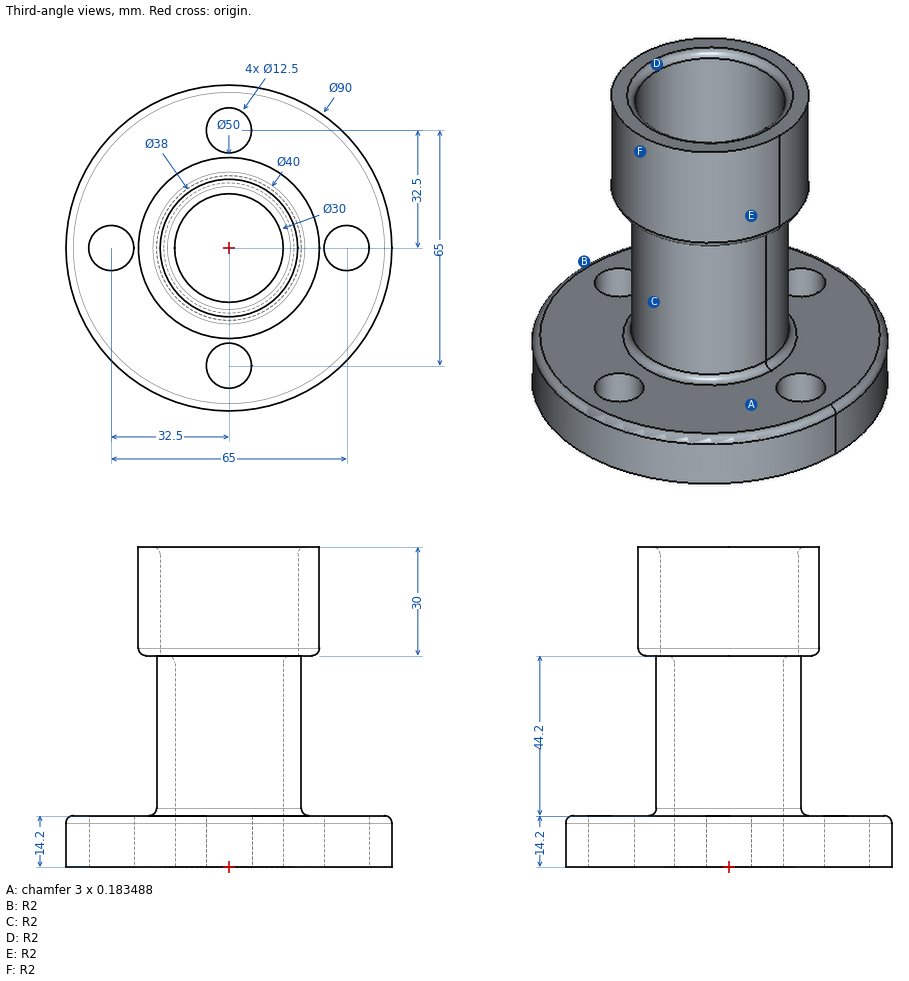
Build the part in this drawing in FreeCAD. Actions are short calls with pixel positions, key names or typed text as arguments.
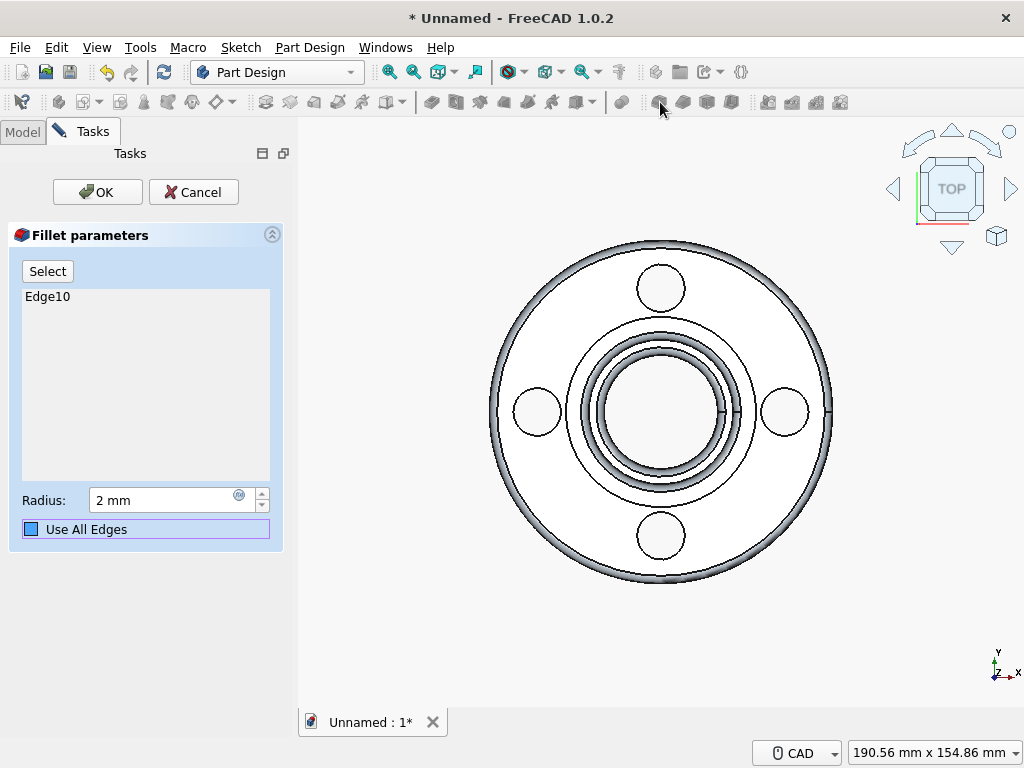
click(98, 192)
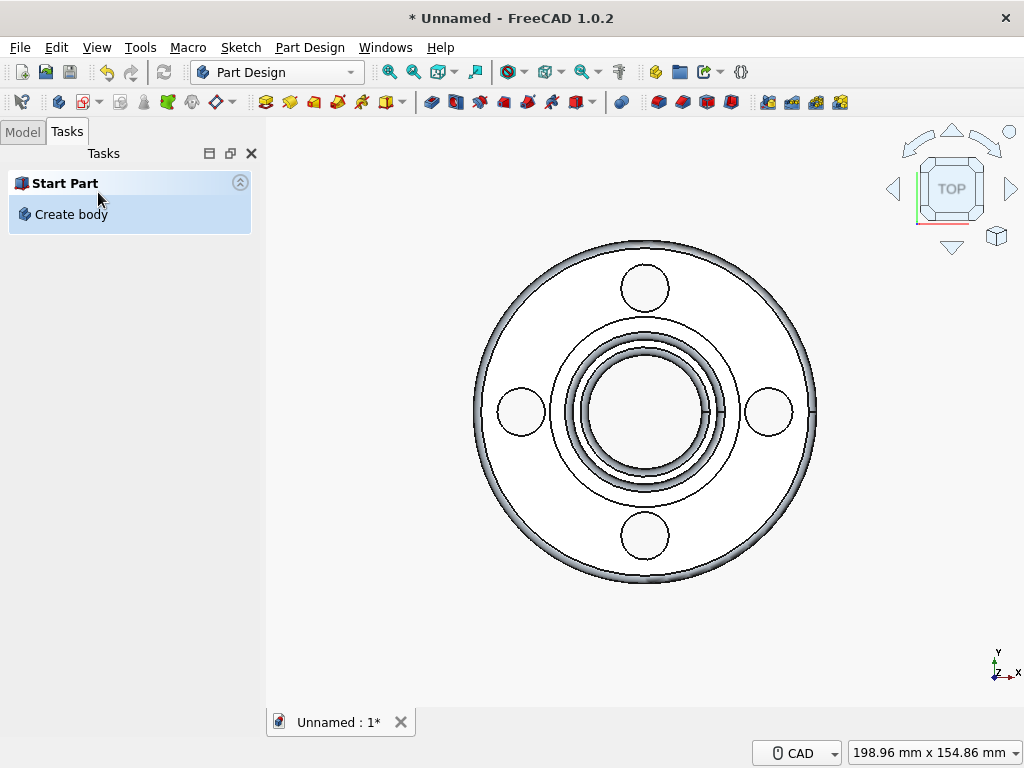
key(0)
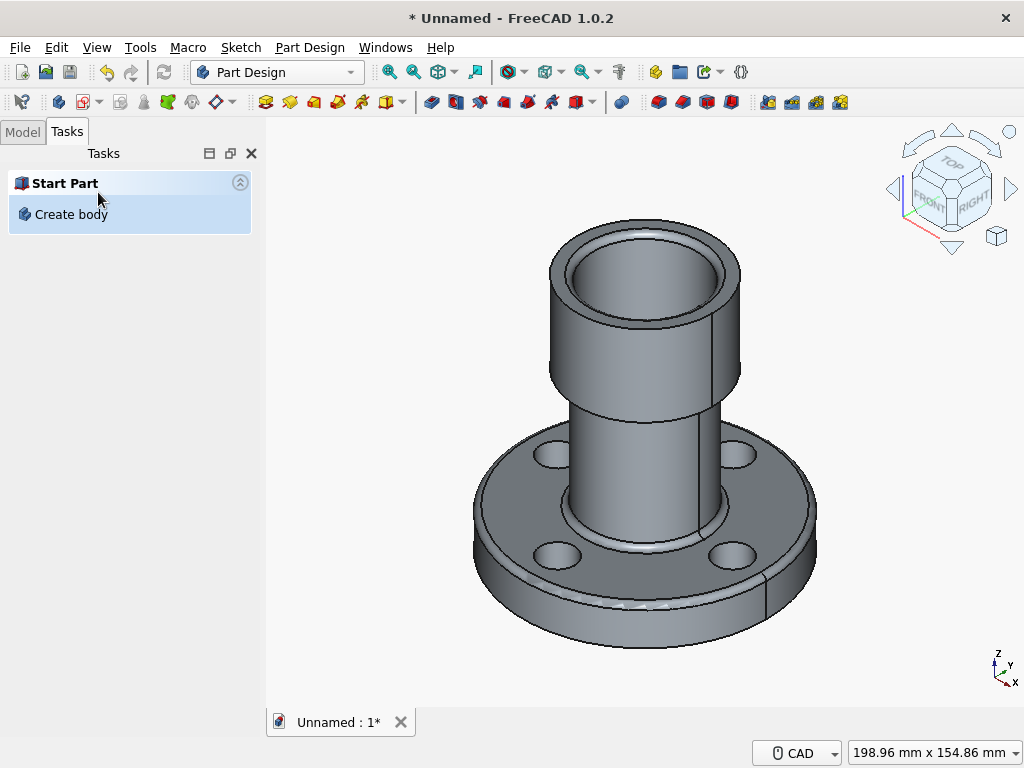
key(2)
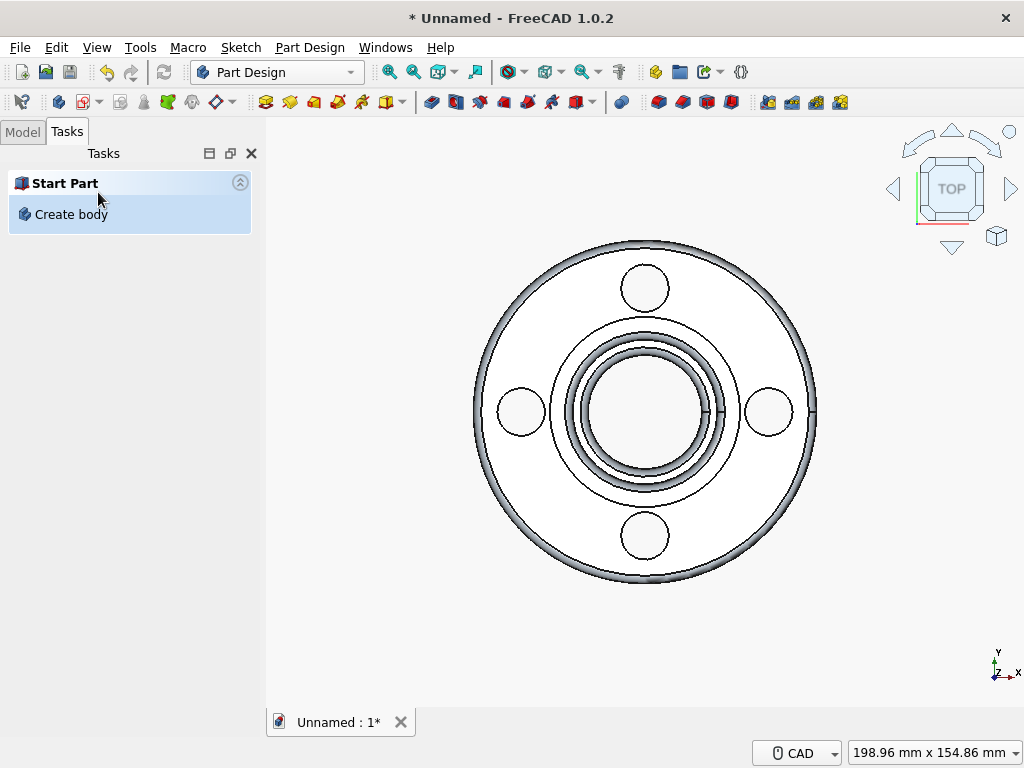
key(1)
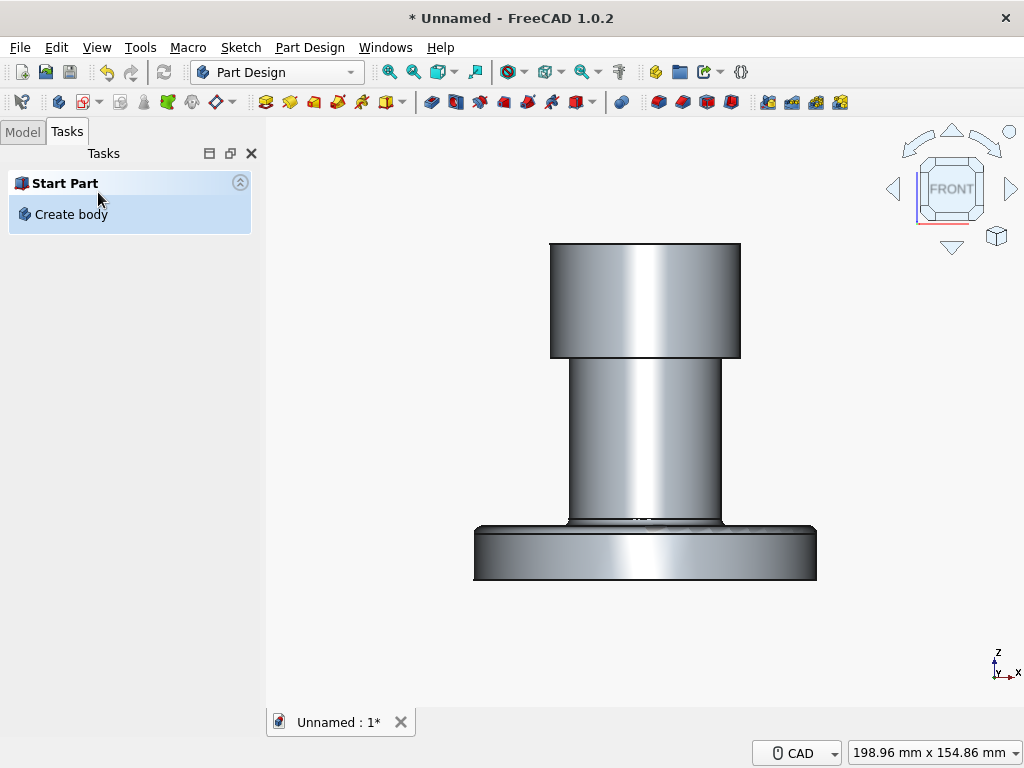
click(568, 357)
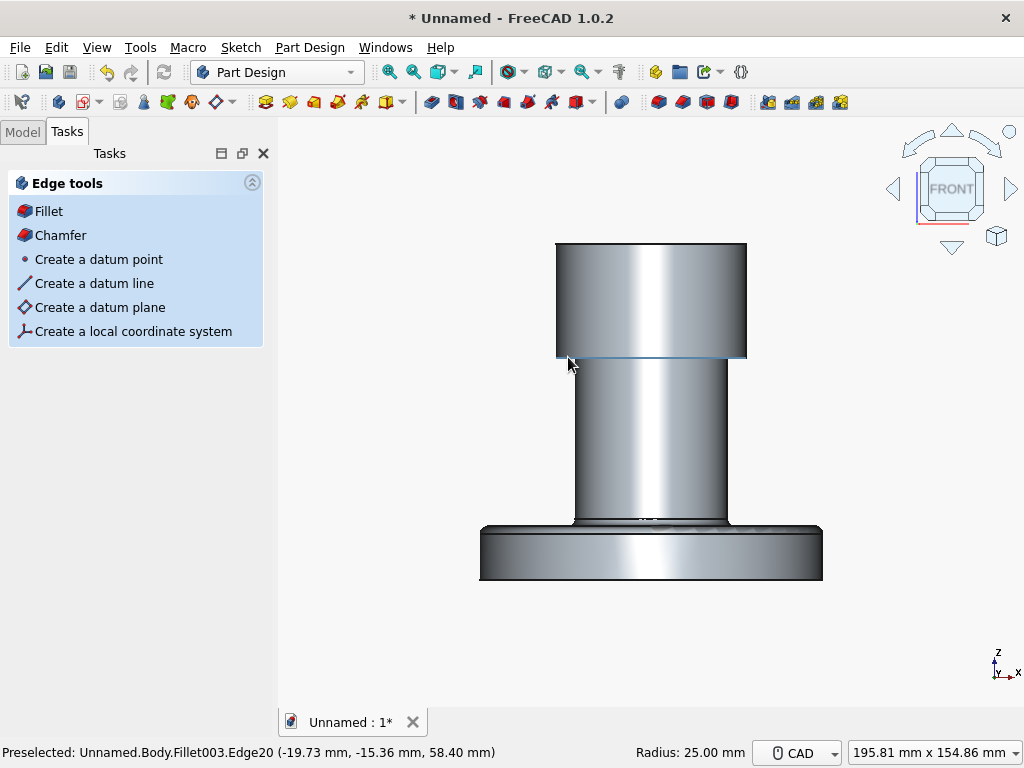
click(660, 102)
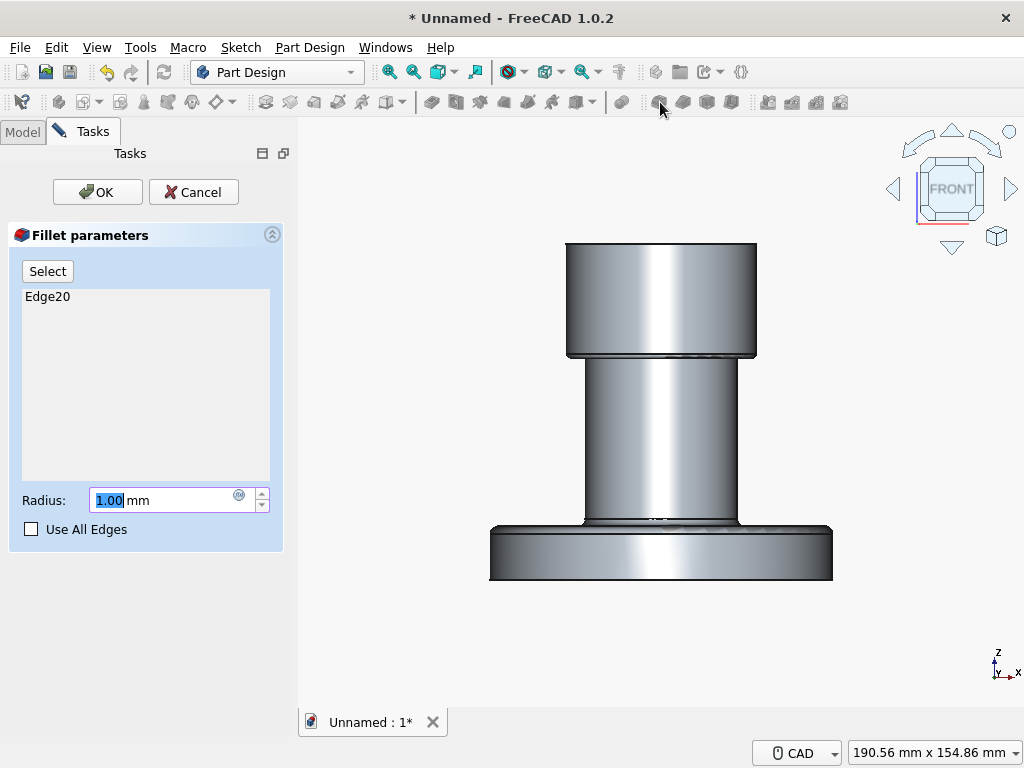
text(2)
key(Tab)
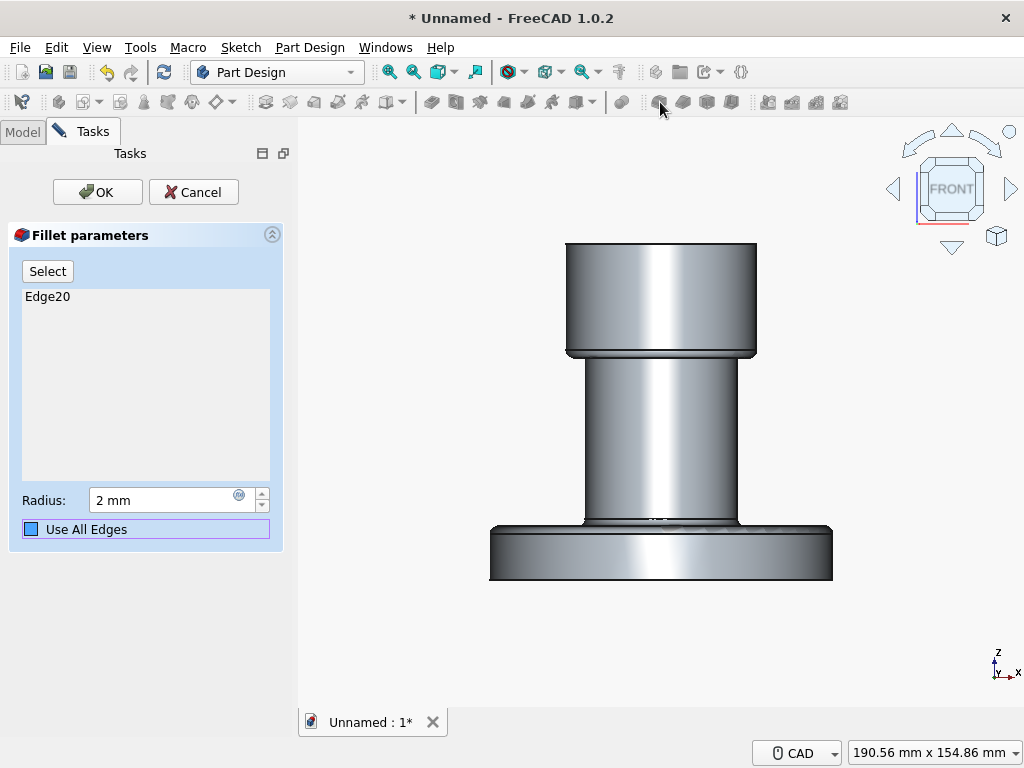
click(98, 192)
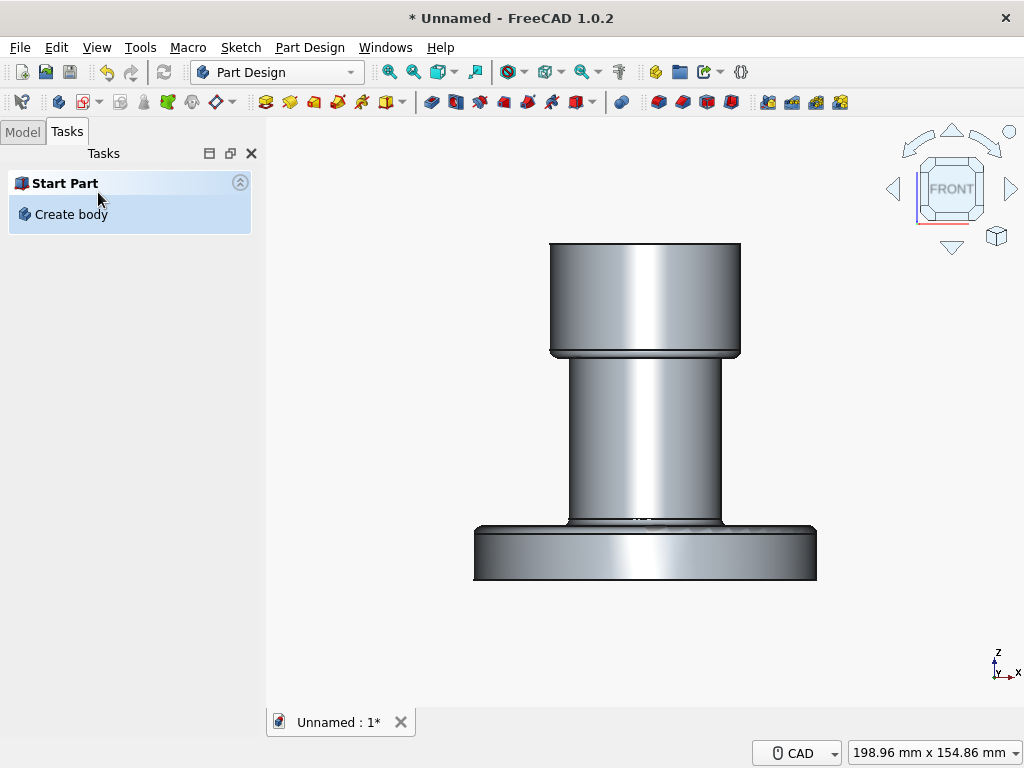
key(0)